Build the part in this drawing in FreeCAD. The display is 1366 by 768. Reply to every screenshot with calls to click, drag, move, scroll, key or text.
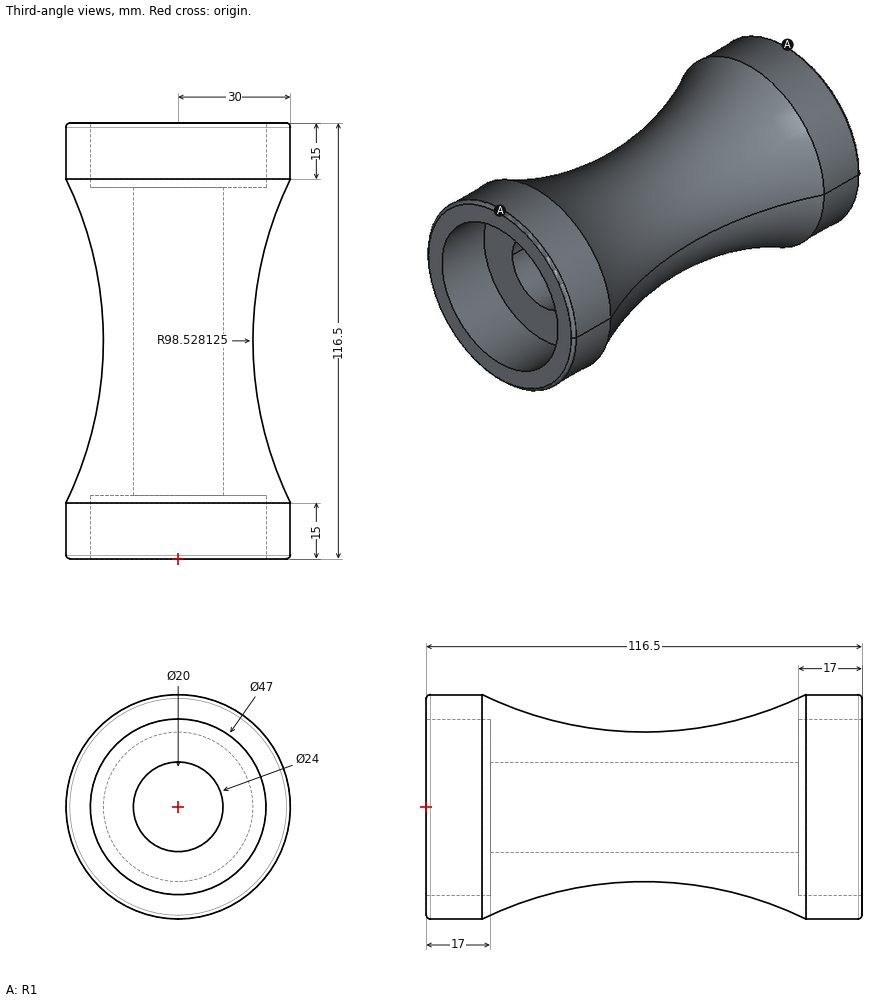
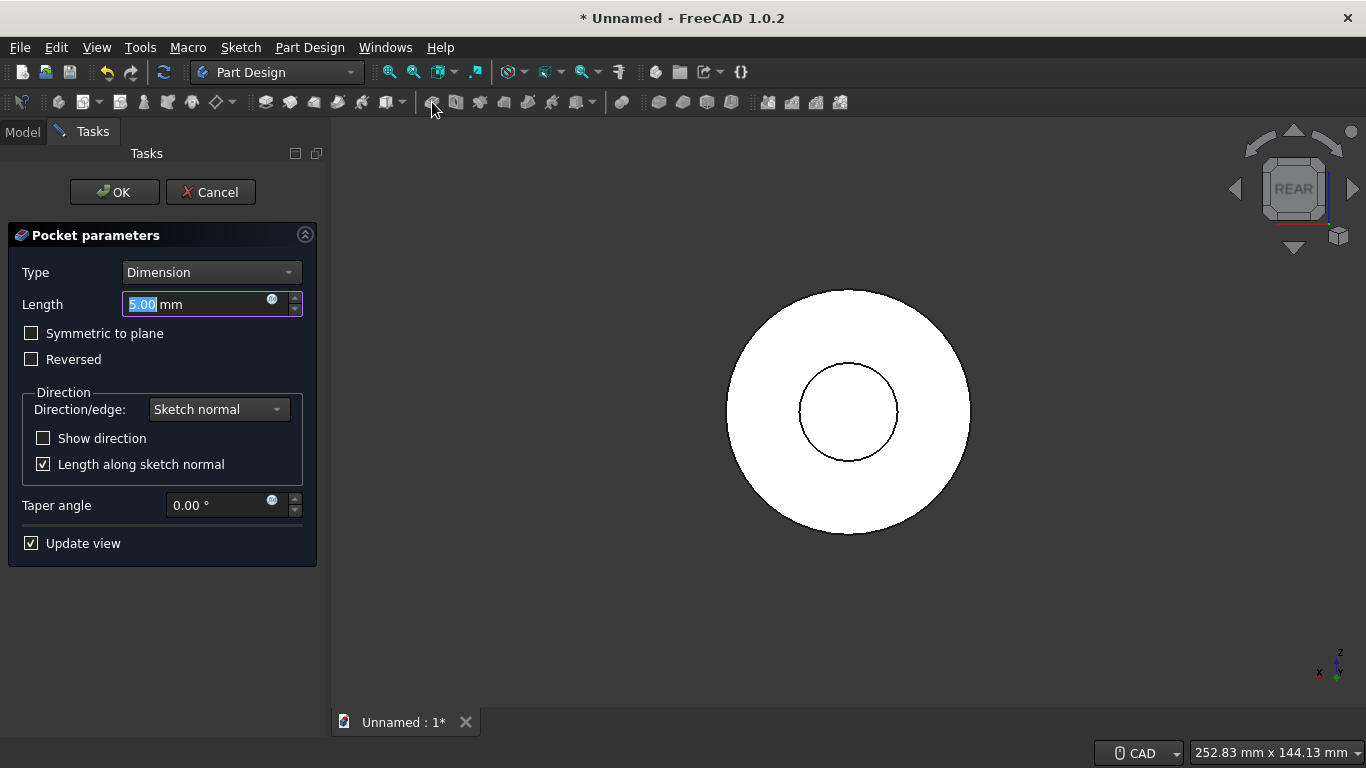
text(116.5)
key(Tab)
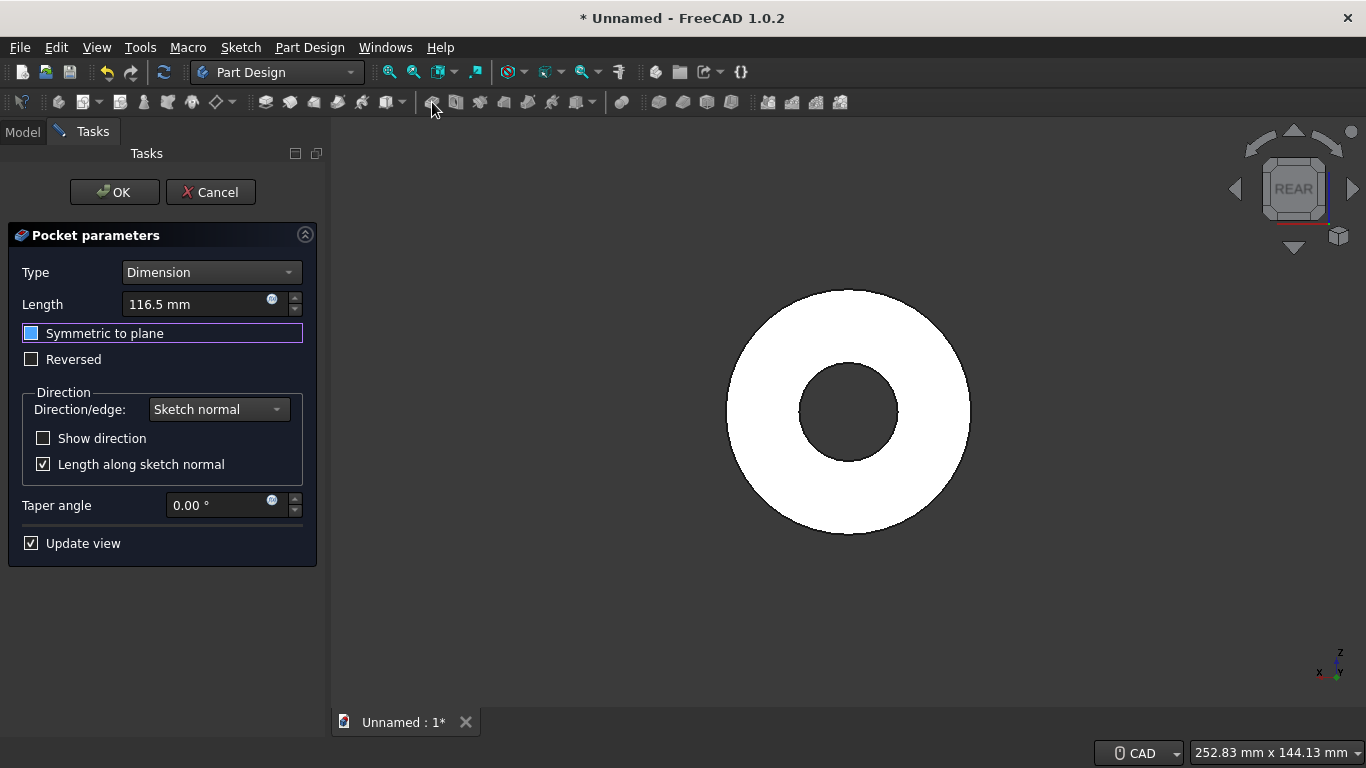
click(115, 192)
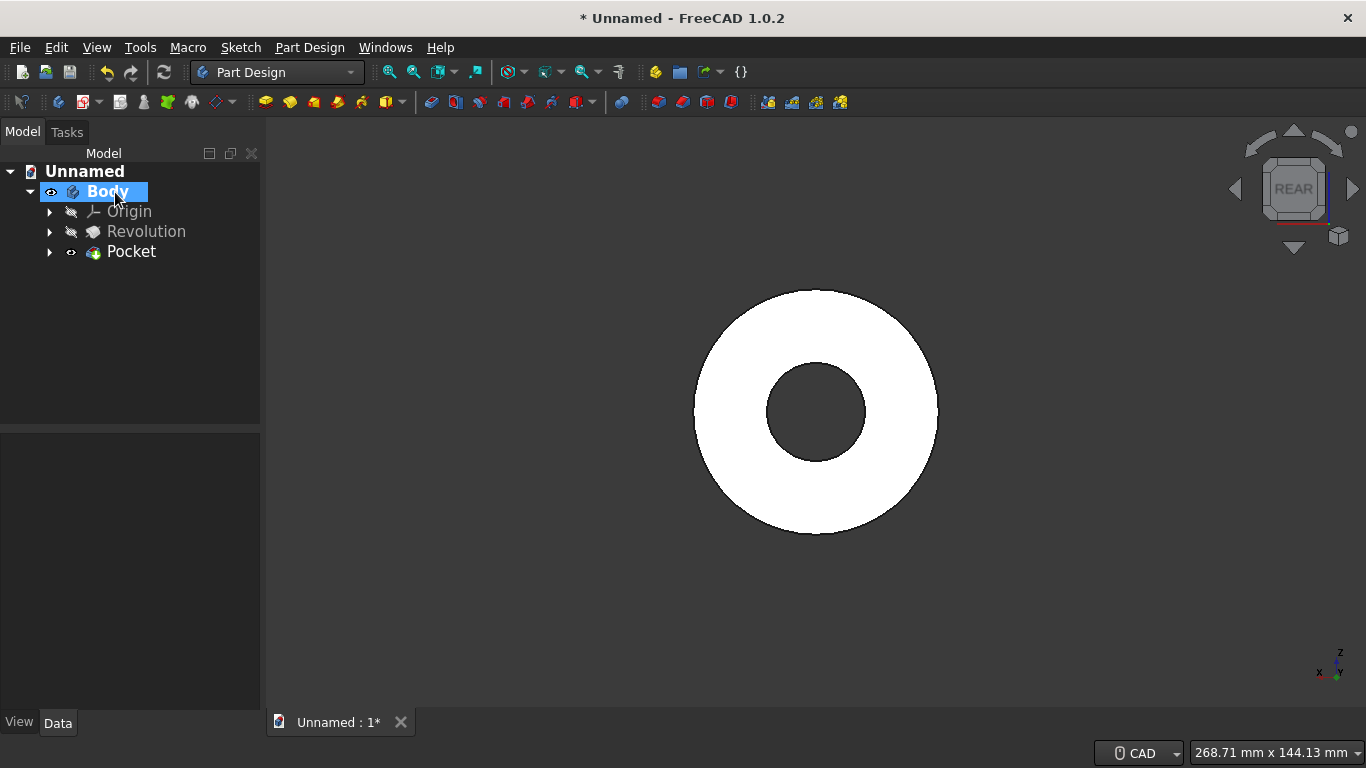
click(390, 72)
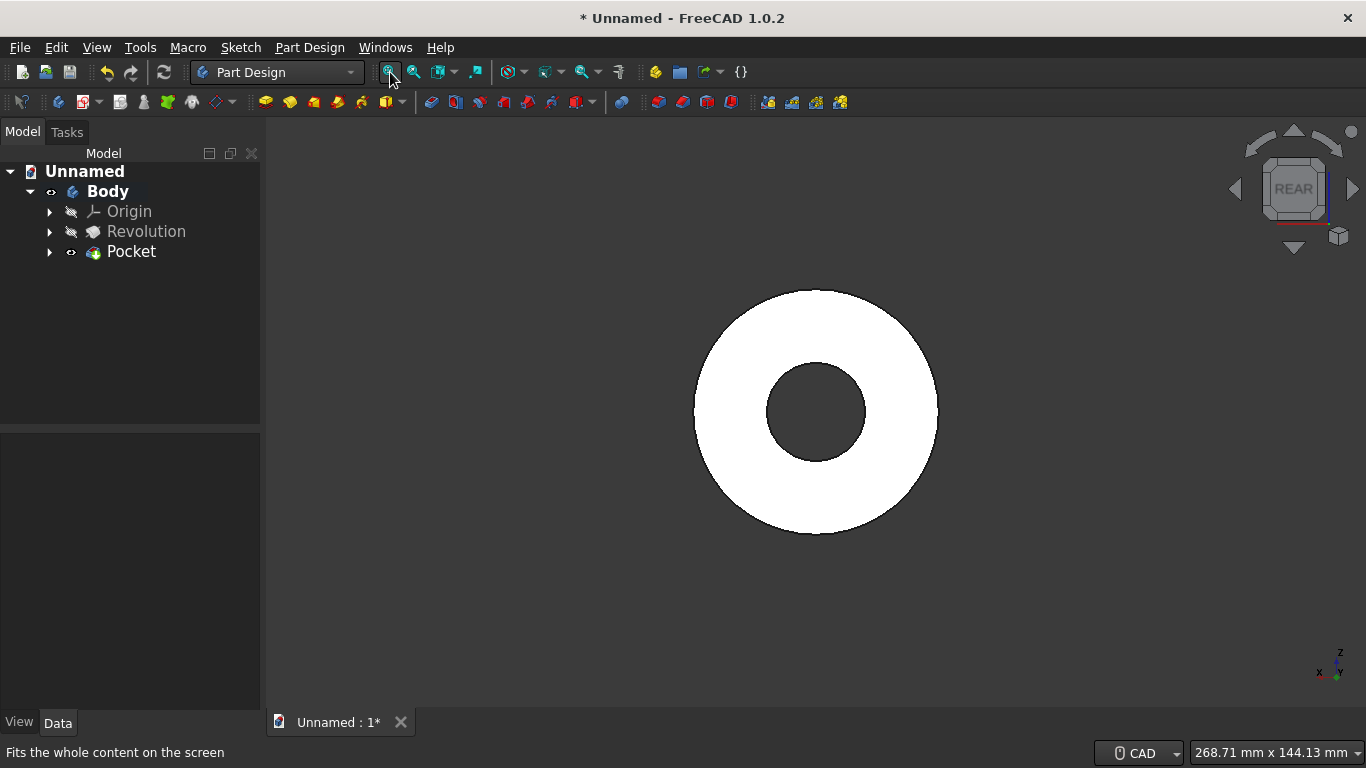
click(851, 341)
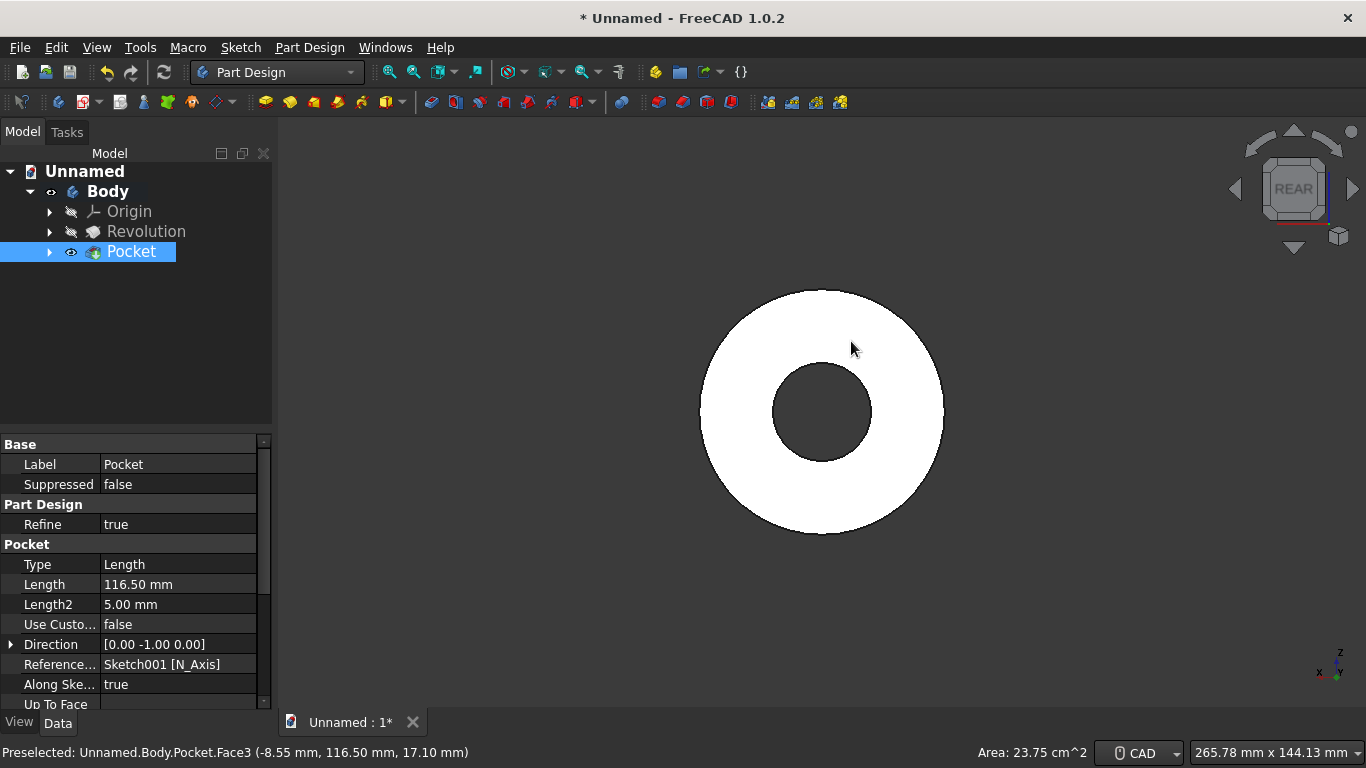
click(84, 102)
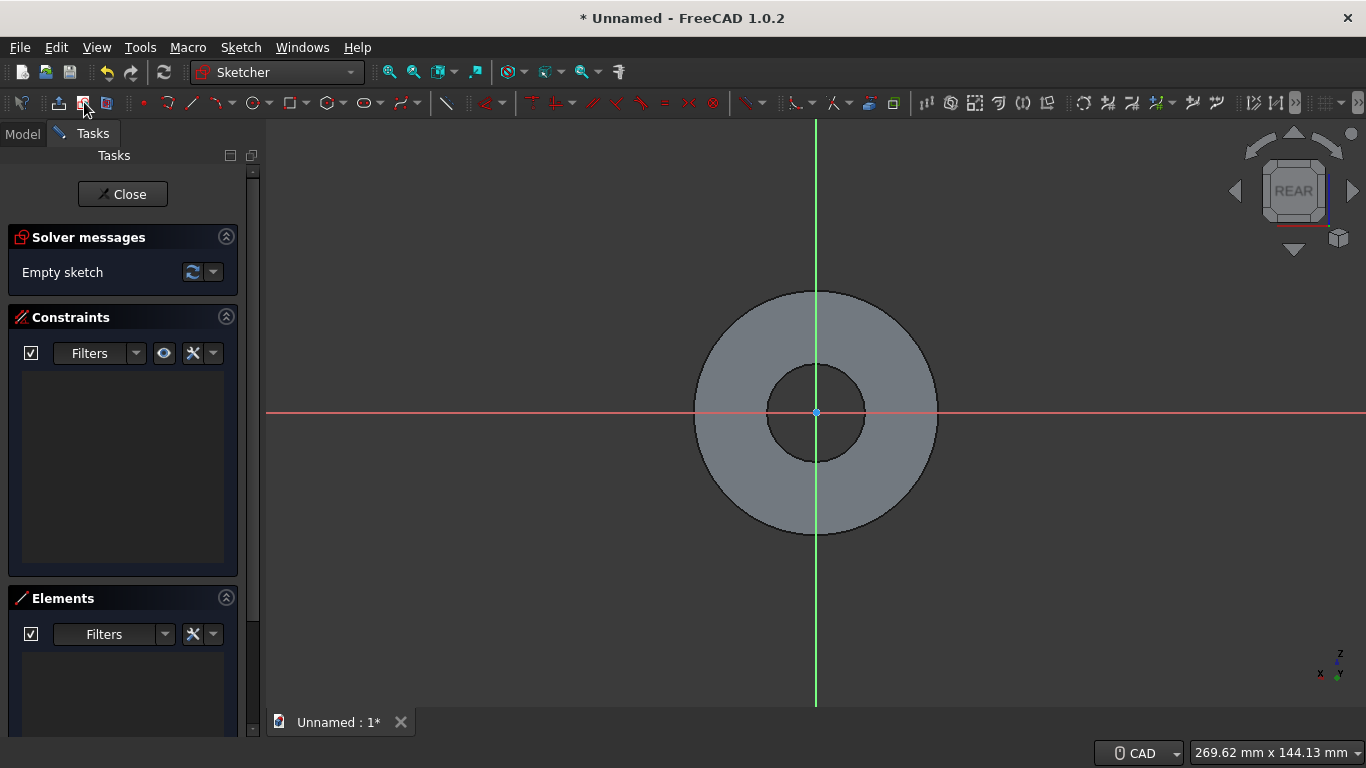
scroll(899, 413, up, 3)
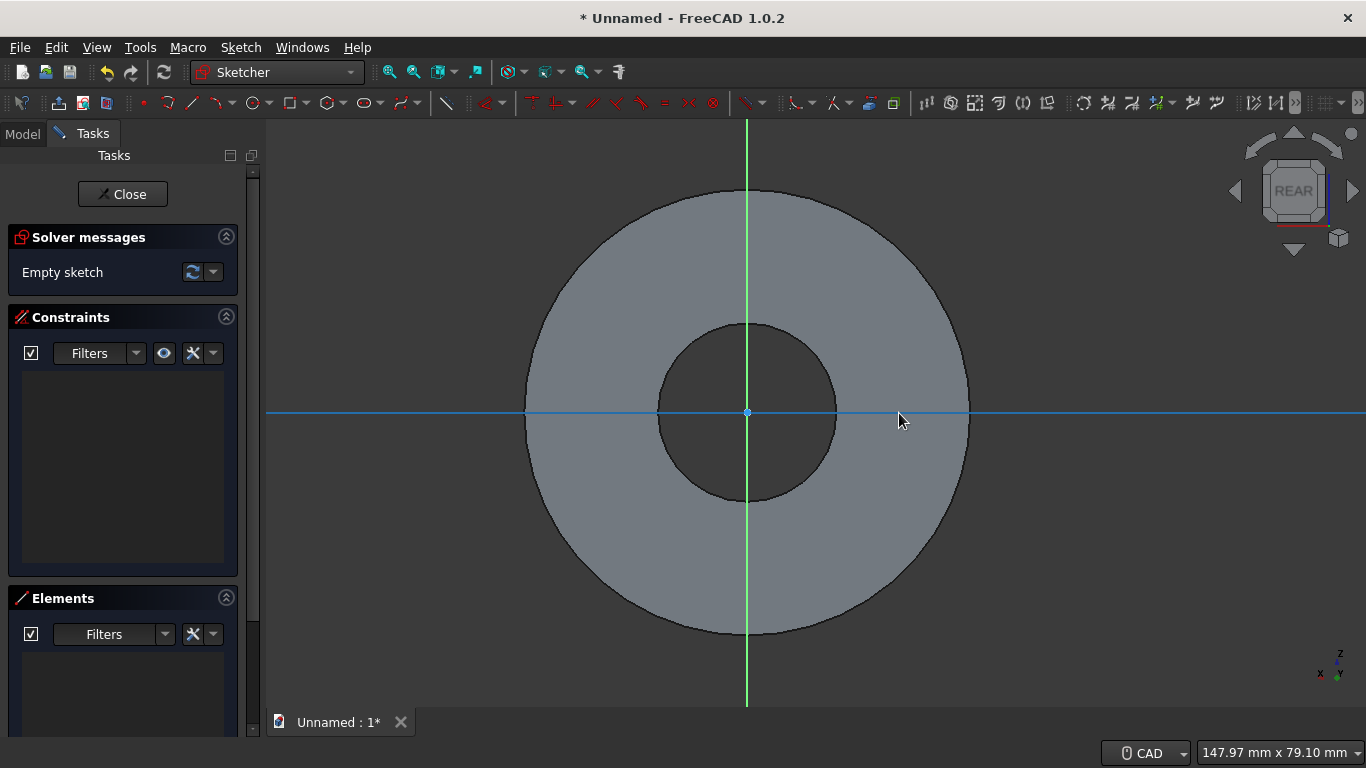
click(254, 104)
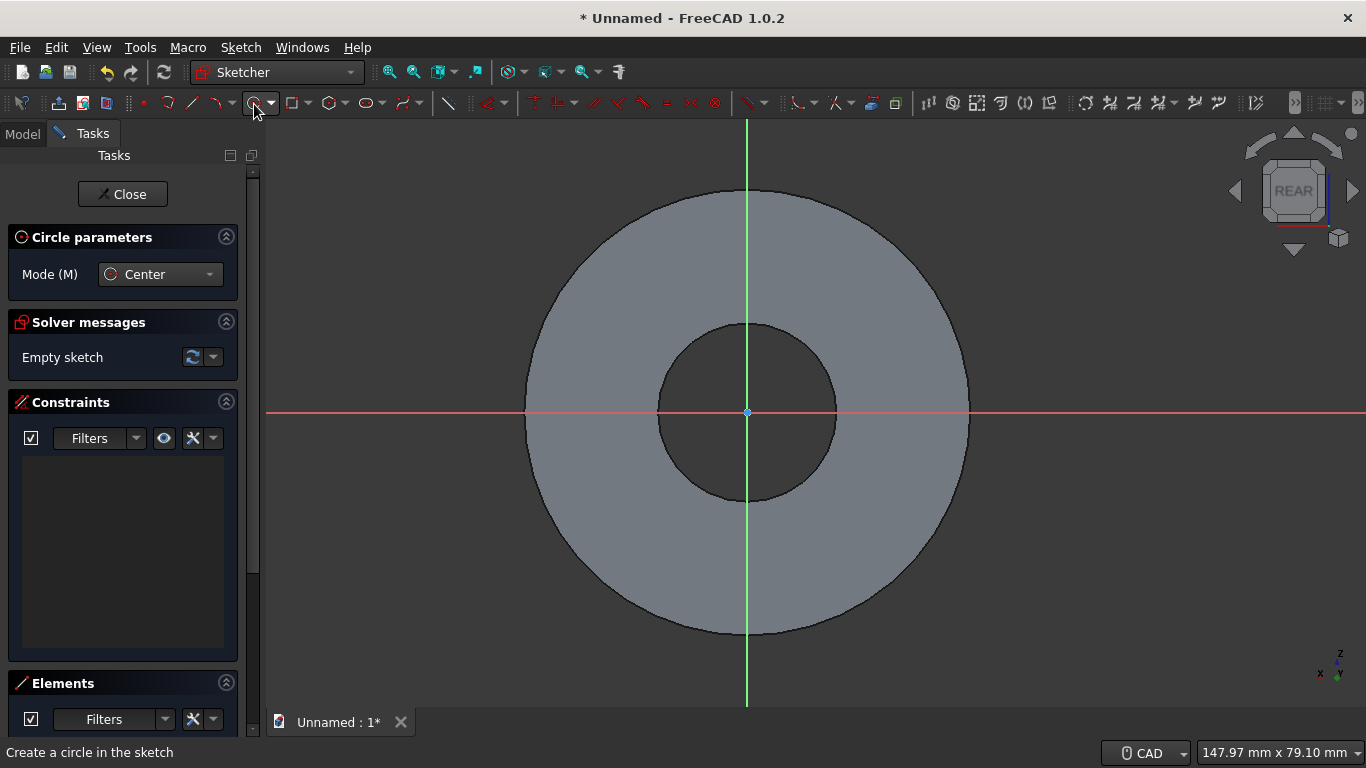
click(747, 413)
click(871, 289)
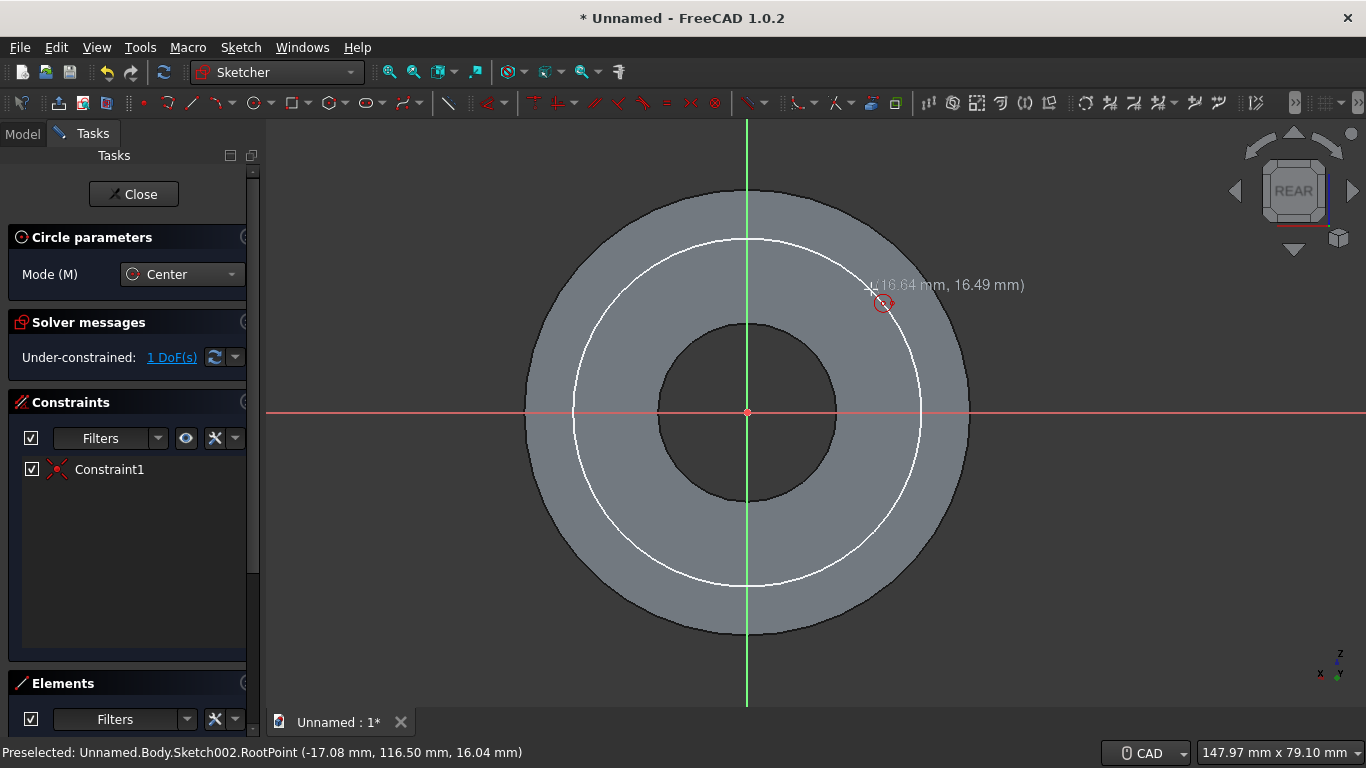
click(747, 413)
click(800, 360)
key(Escape)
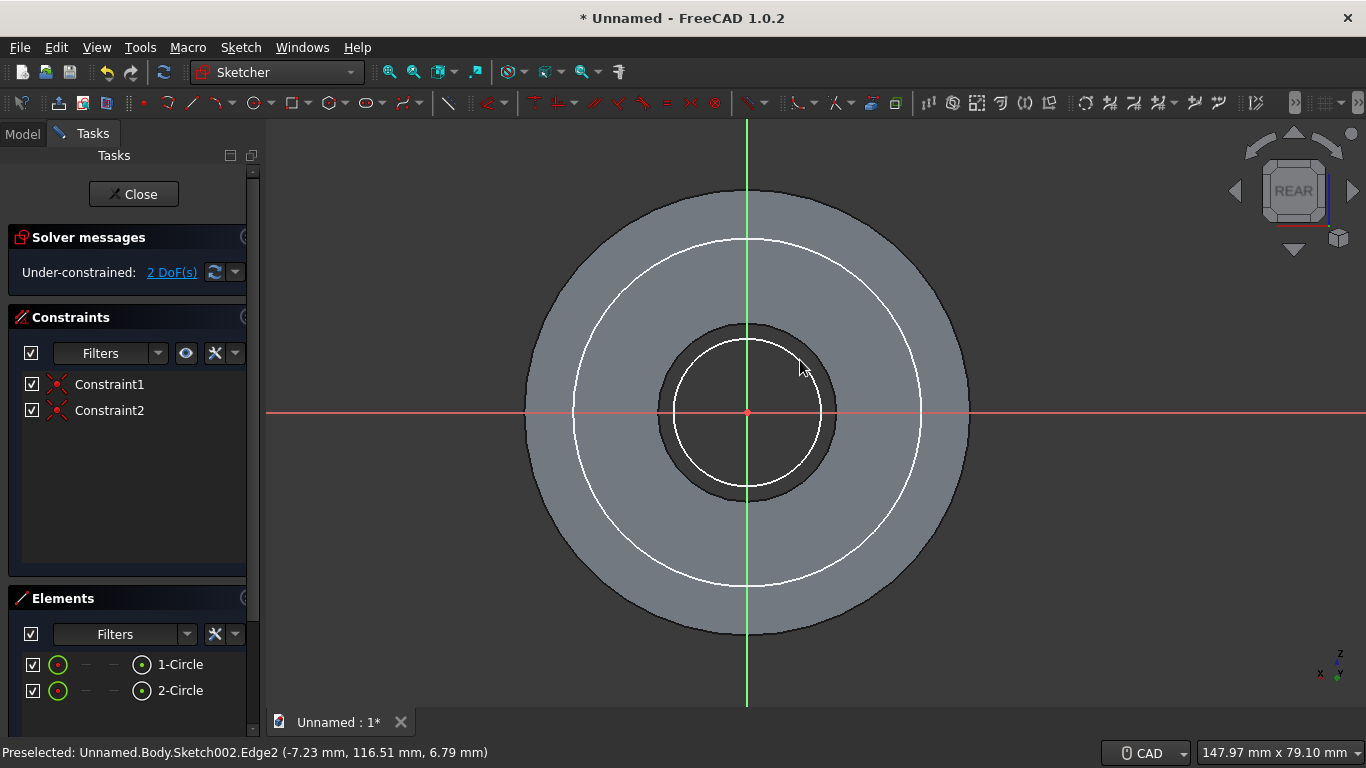
click(488, 104)